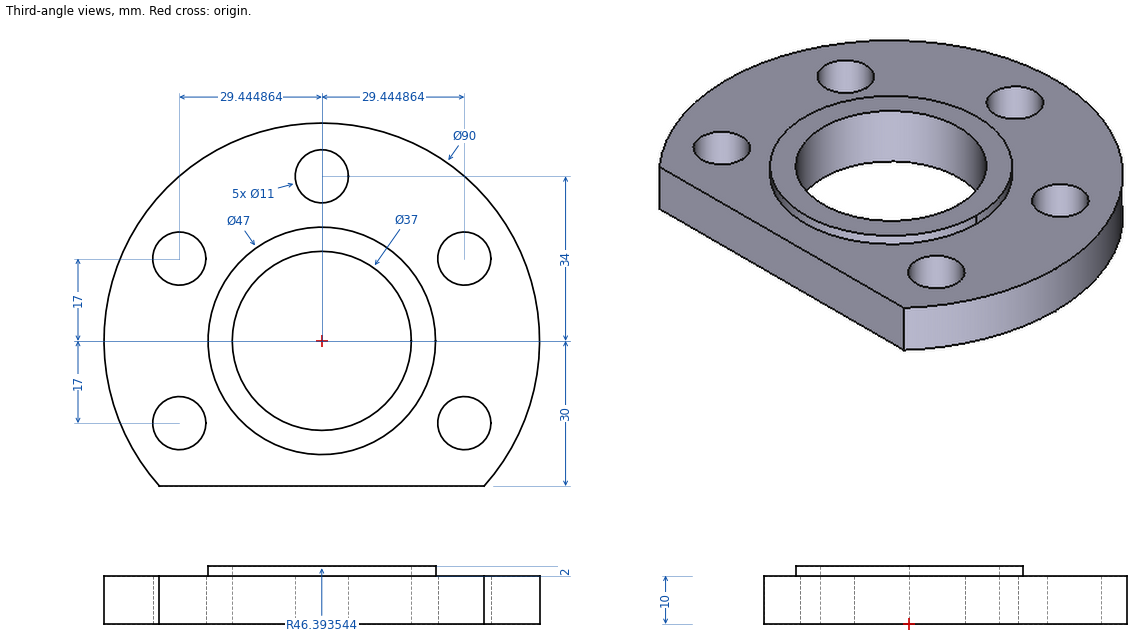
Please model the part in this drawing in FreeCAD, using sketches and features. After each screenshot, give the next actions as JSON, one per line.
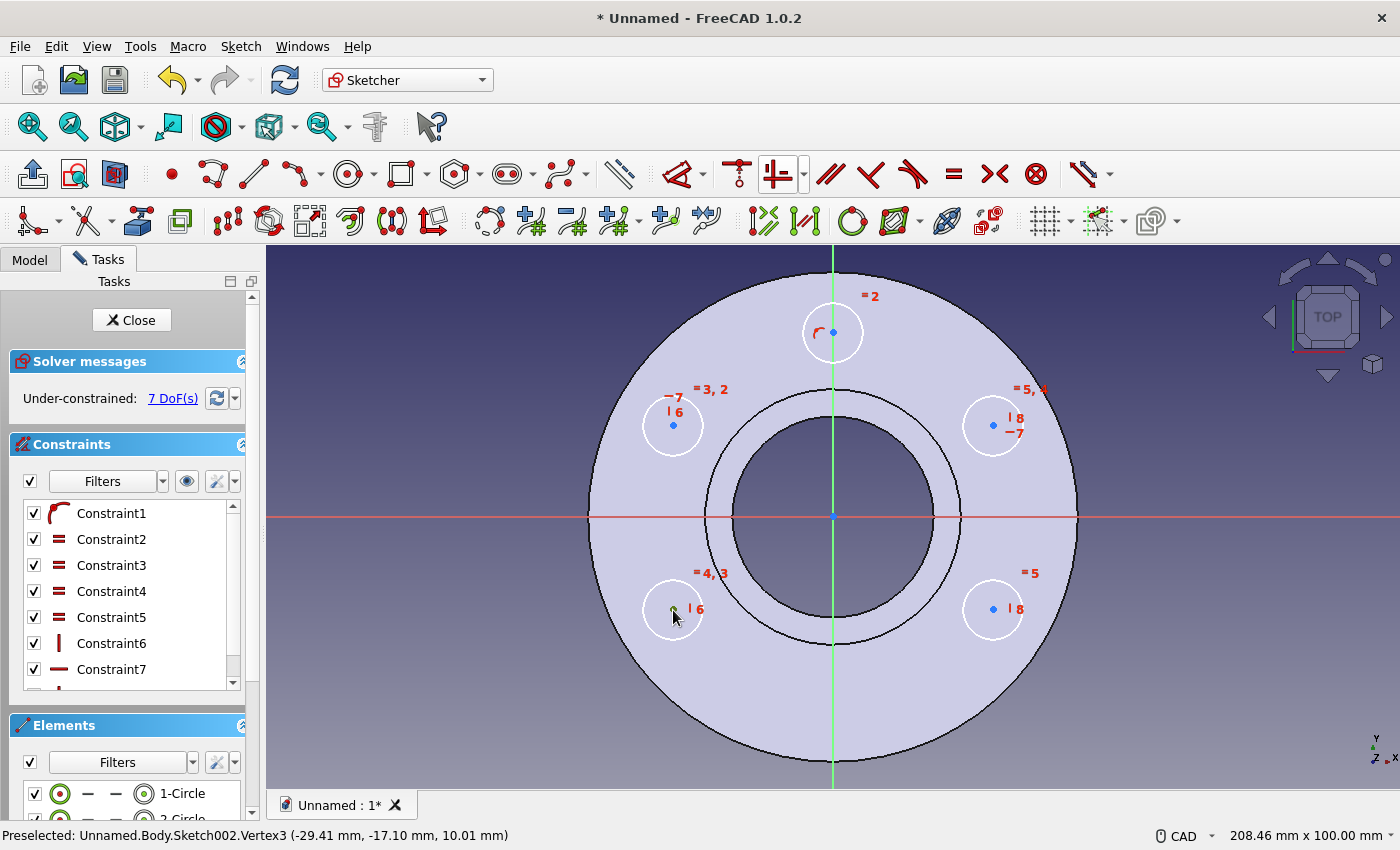
{"action": "left_click", "coordinate": [993, 610]}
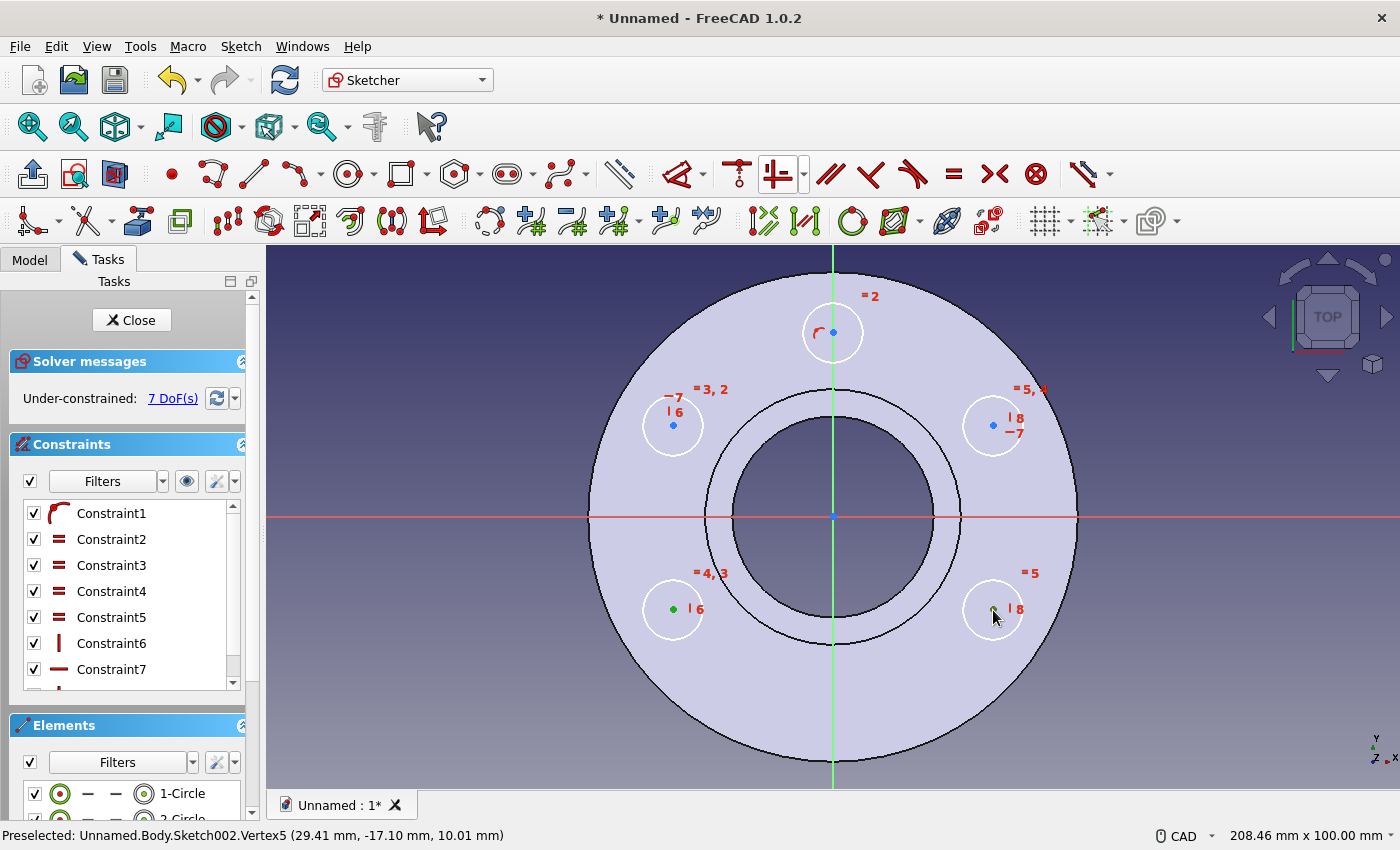
{"action": "key", "text": "h"}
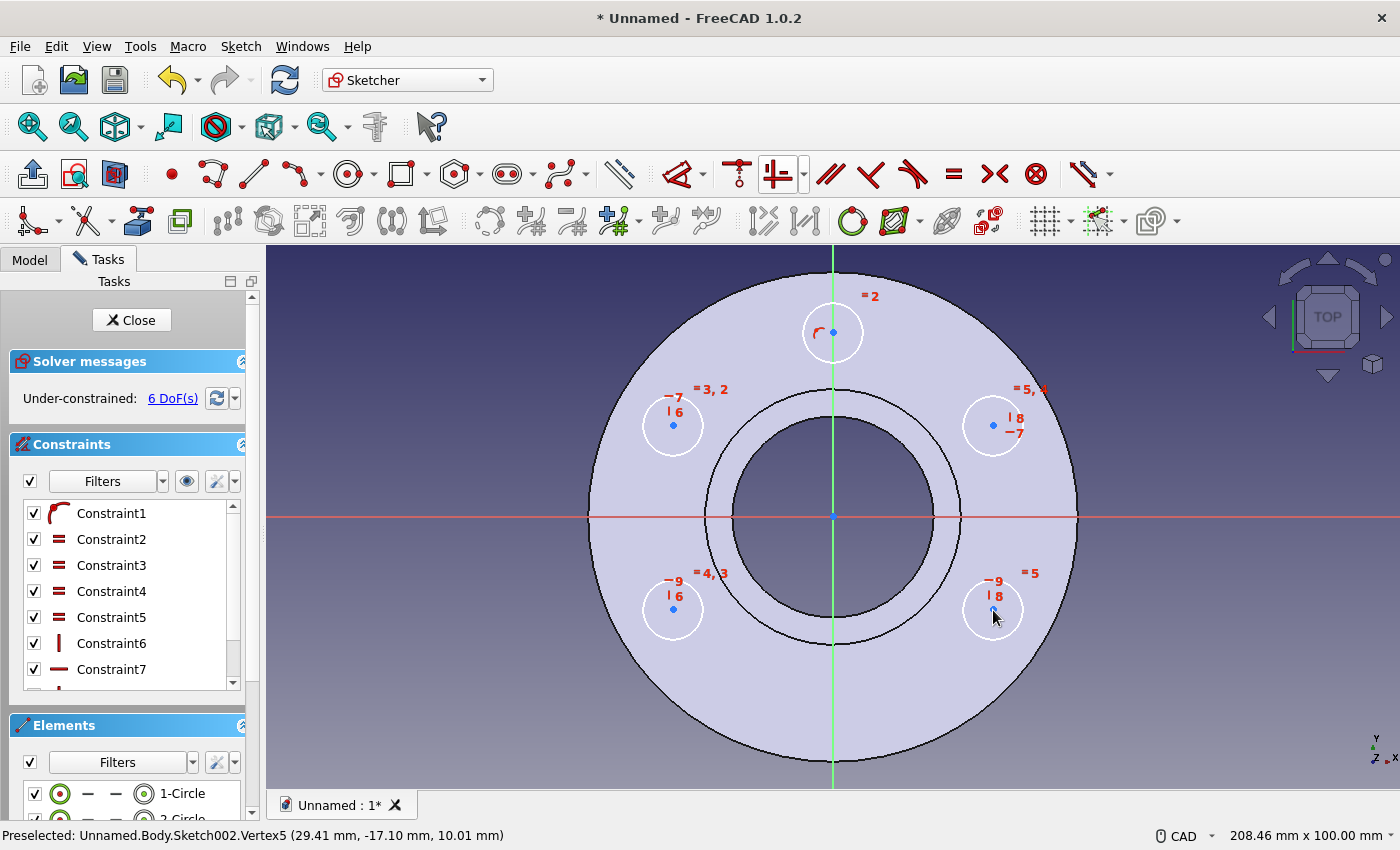
{"action": "left_click", "coordinate": [676, 174]}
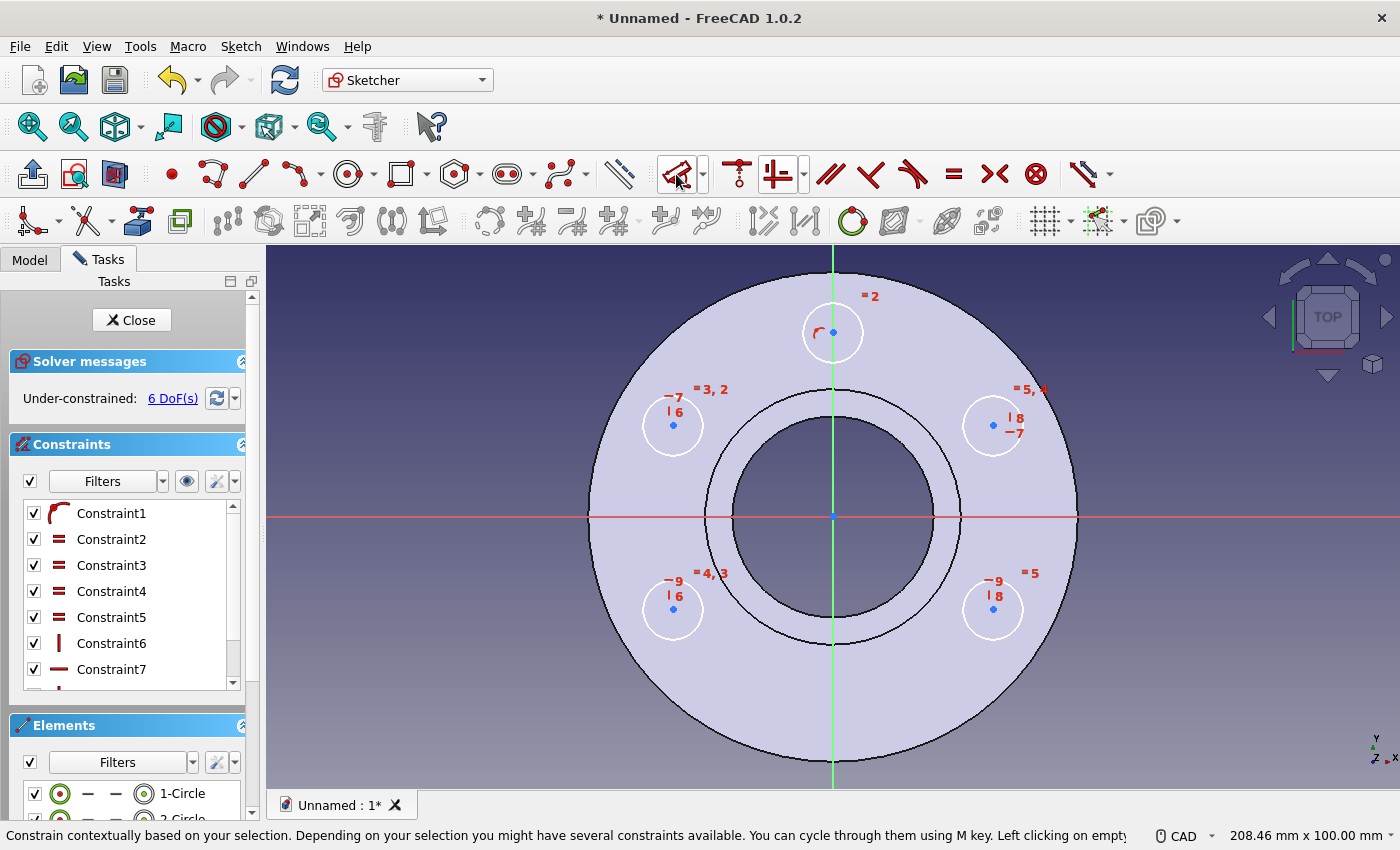
{"action": "left_click", "coordinate": [854, 312]}
{"action": "left_click", "coordinate": [877, 289]}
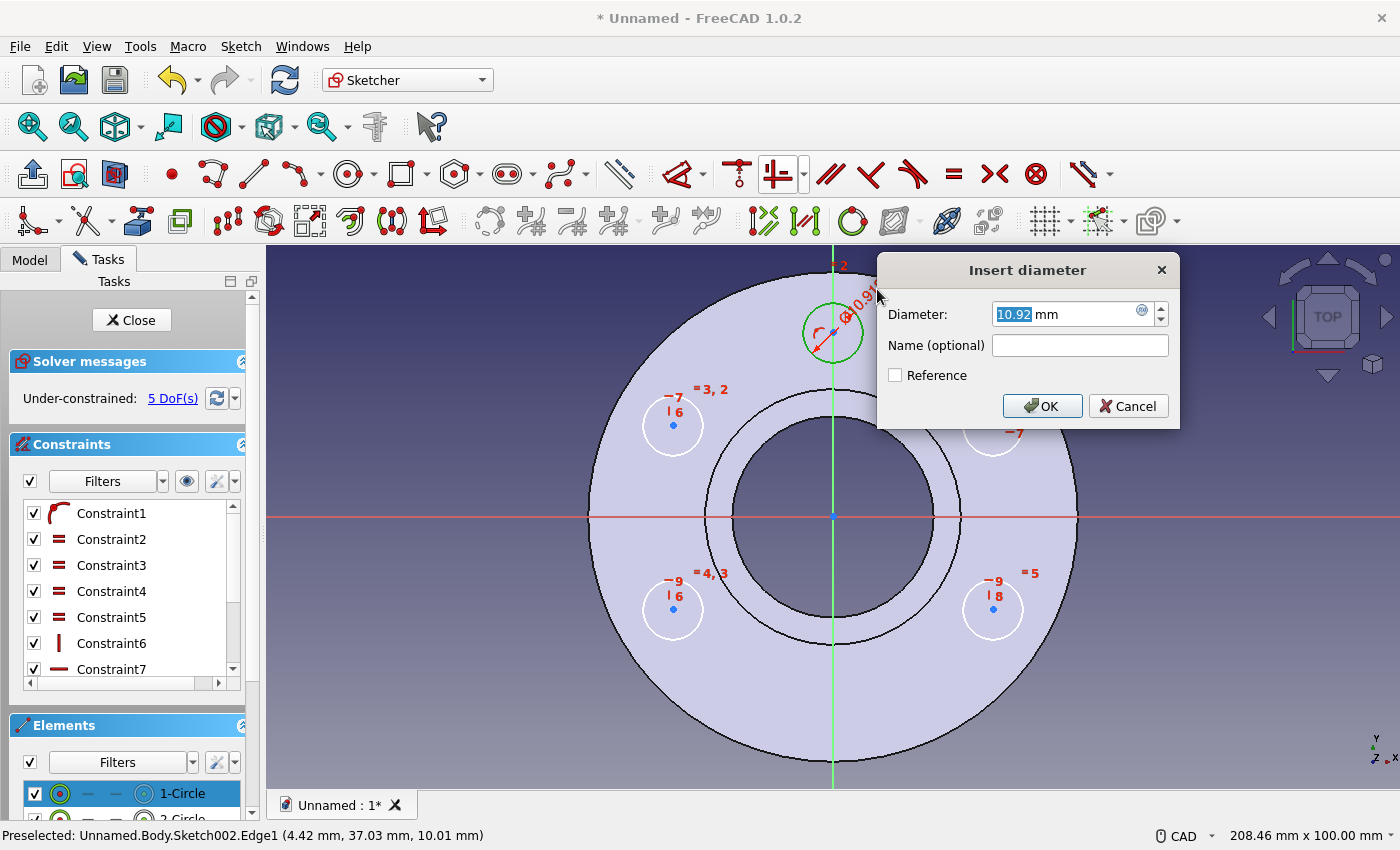
{"action": "type", "text": "11"}
{"action": "key", "text": "Return"}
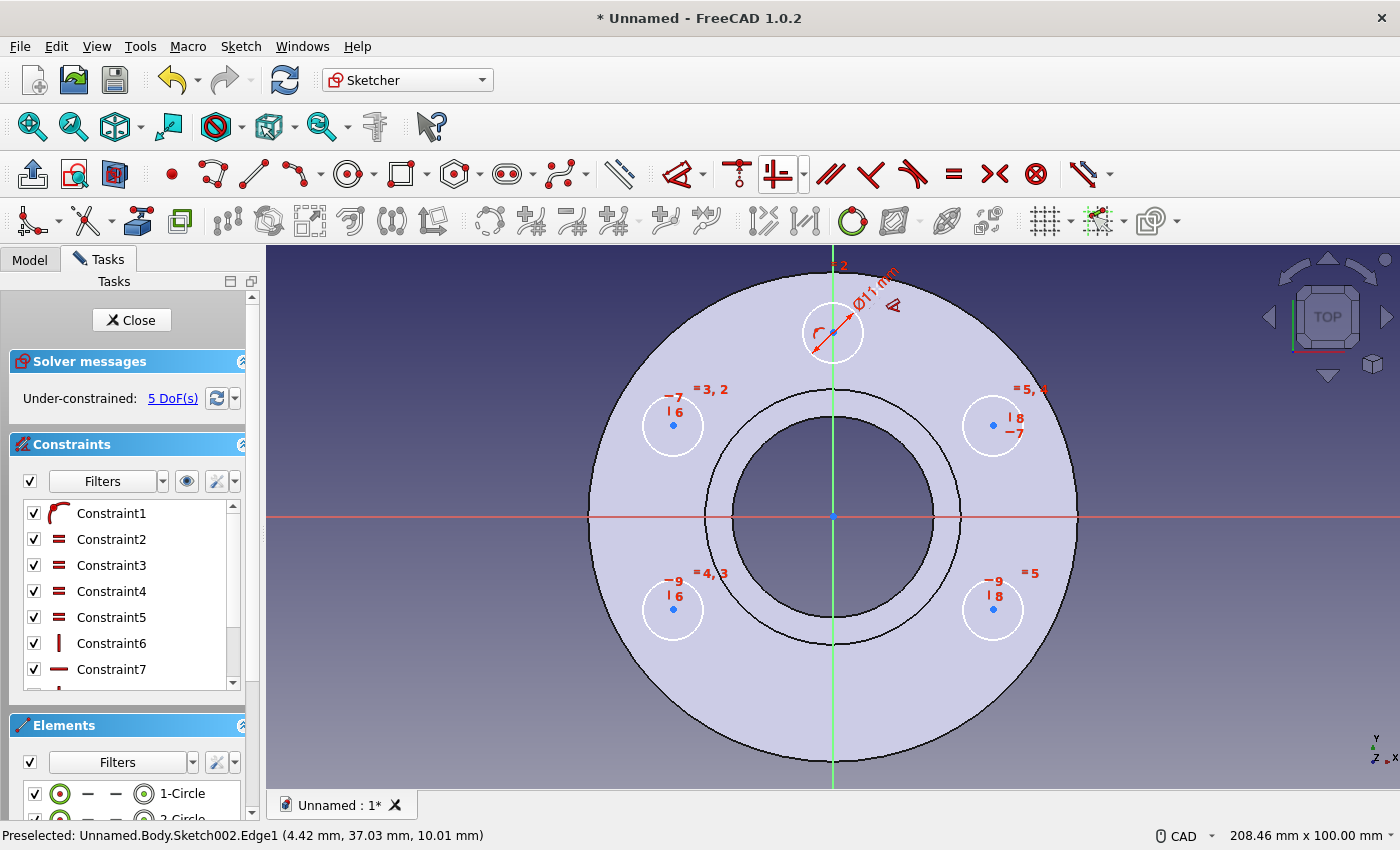
{"action": "left_click", "coordinate": [833, 333]}
{"action": "left_click", "coordinate": [867, 425]}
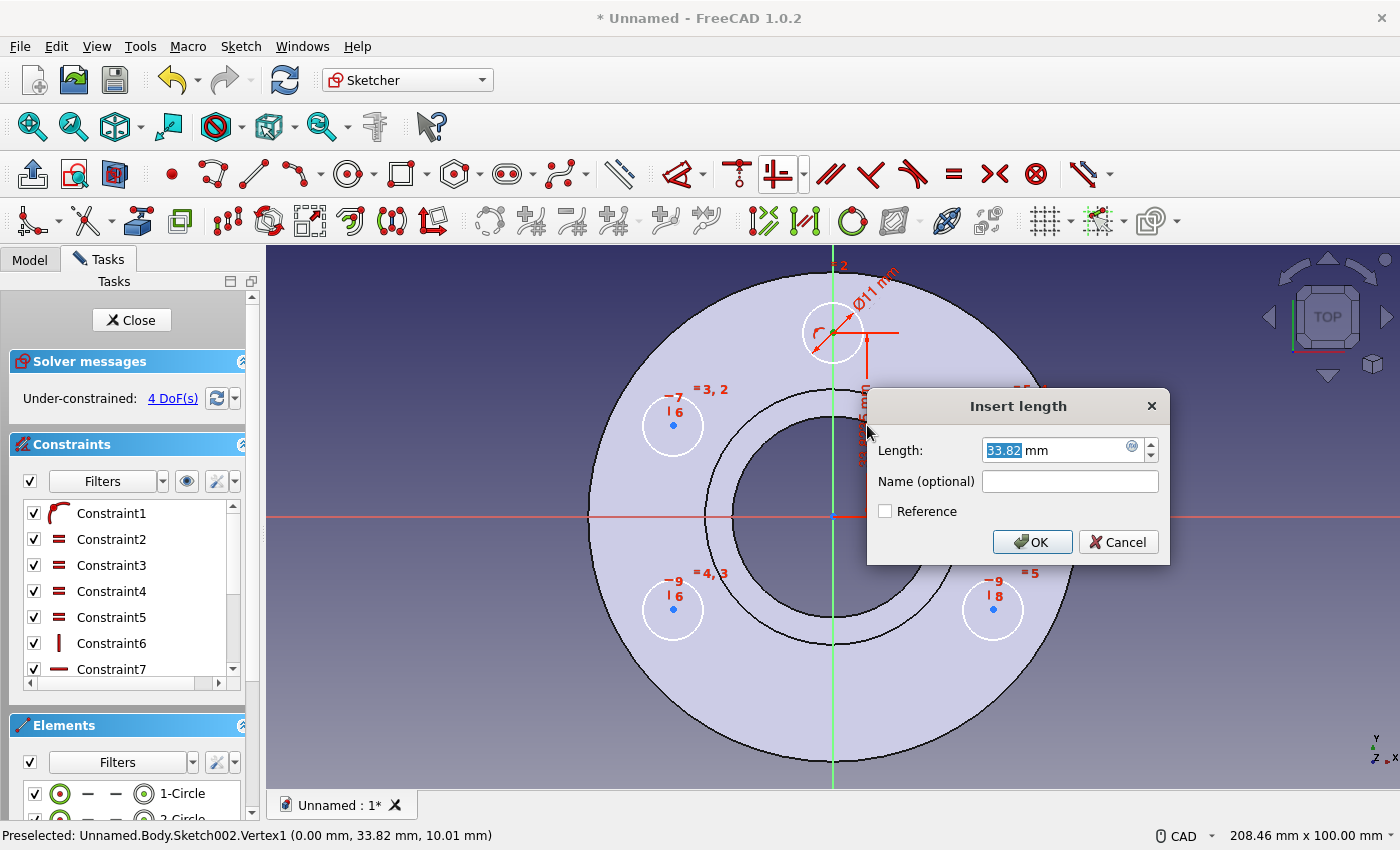
{"action": "type", "text": "34"}
{"action": "key", "text": "Return"}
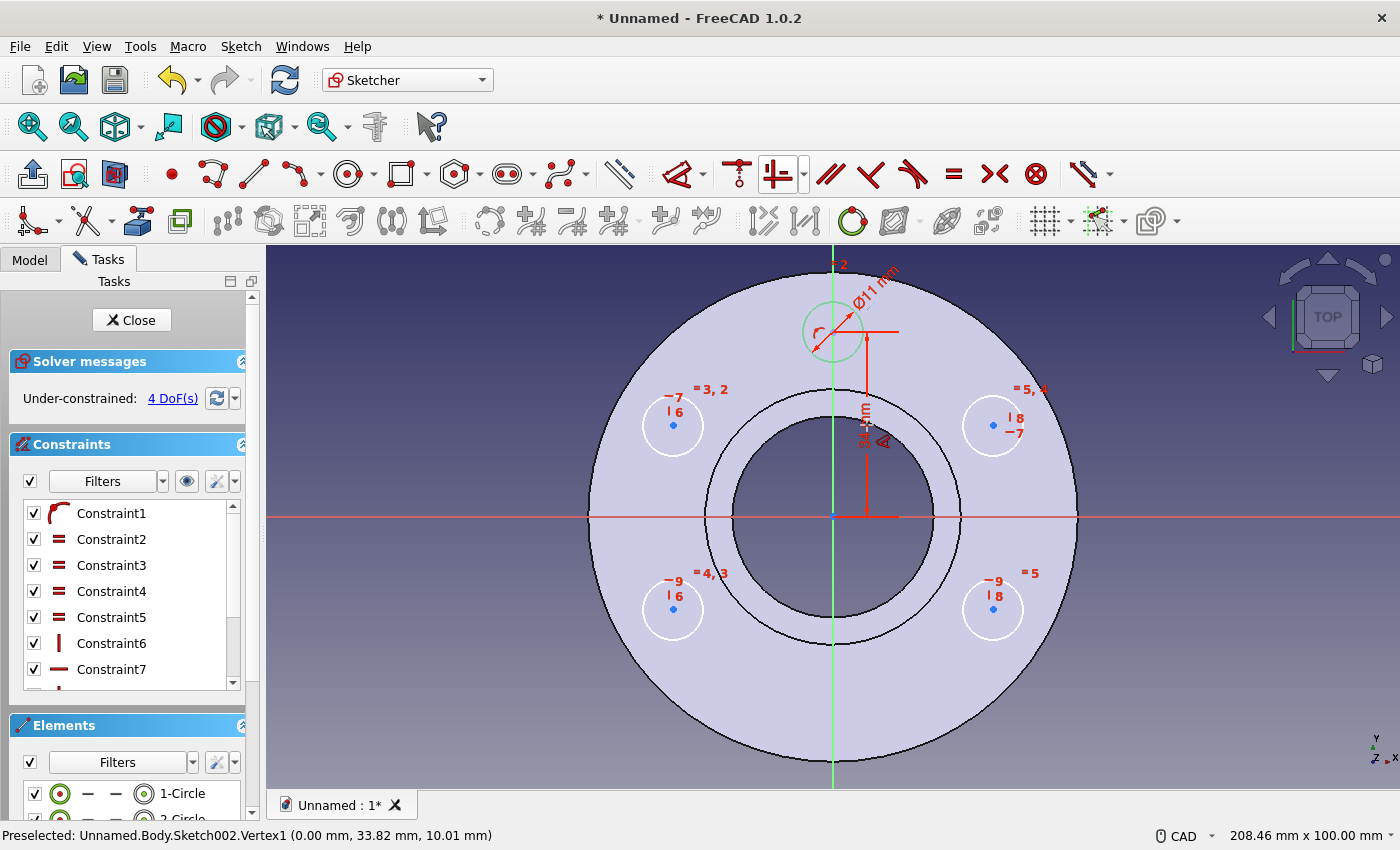
{"action": "left_click", "coordinate": [673, 426]}
{"action": "left_click", "coordinate": [639, 471]}